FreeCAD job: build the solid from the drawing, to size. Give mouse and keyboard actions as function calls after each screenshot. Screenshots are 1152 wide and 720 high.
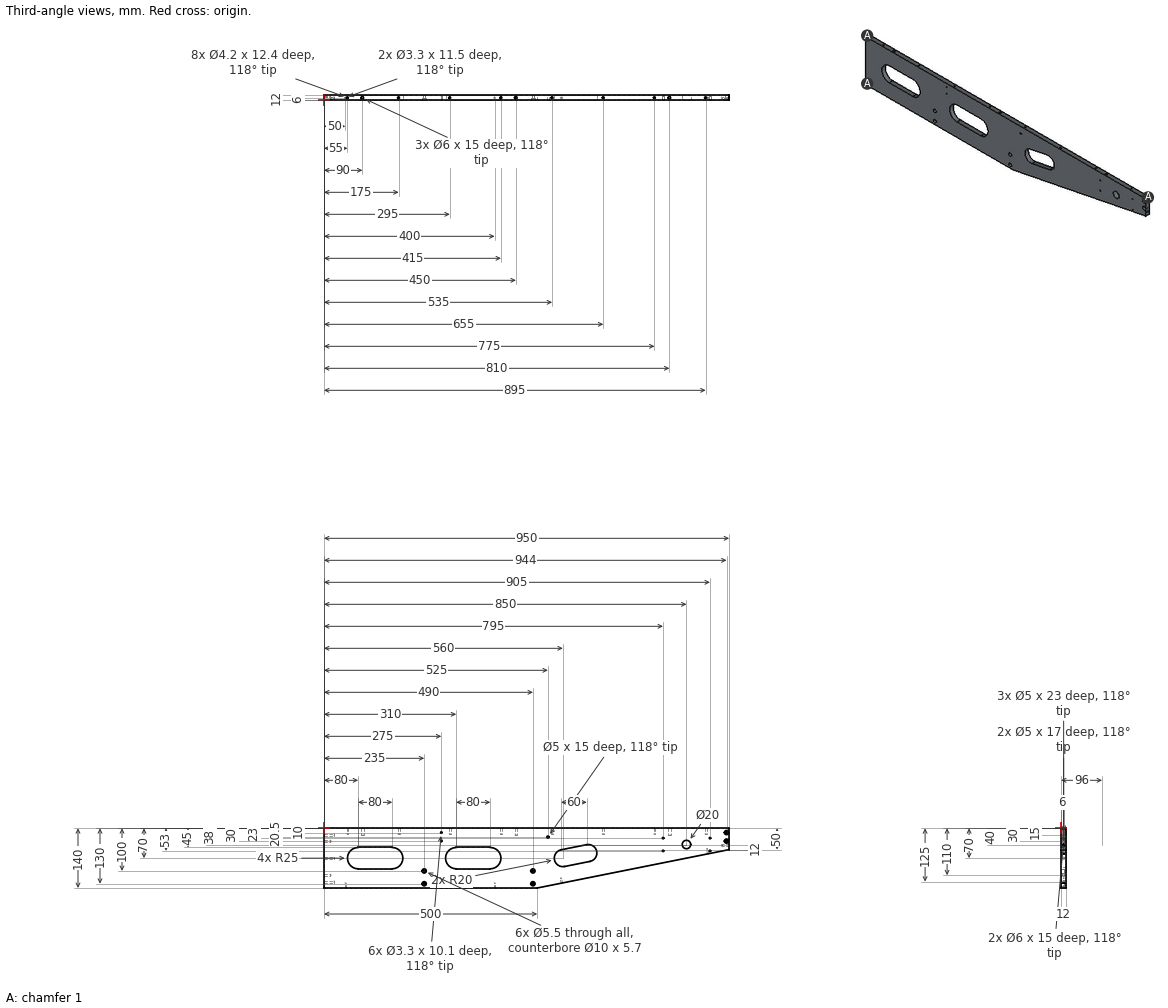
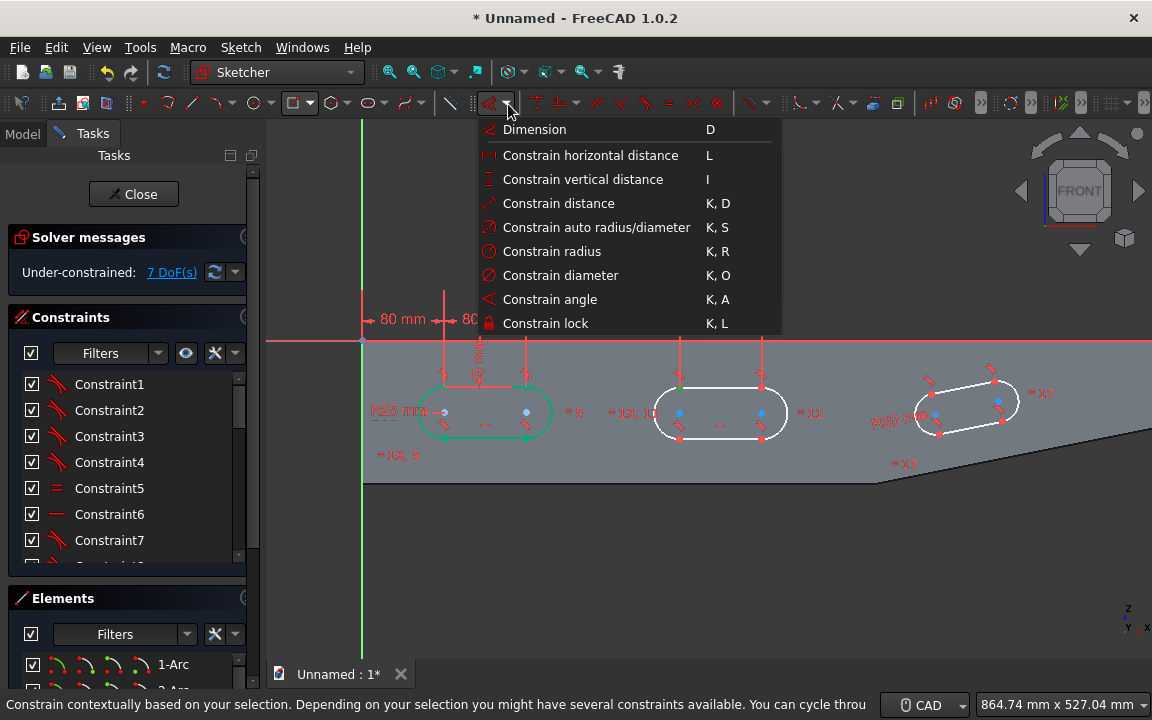
click(630, 179)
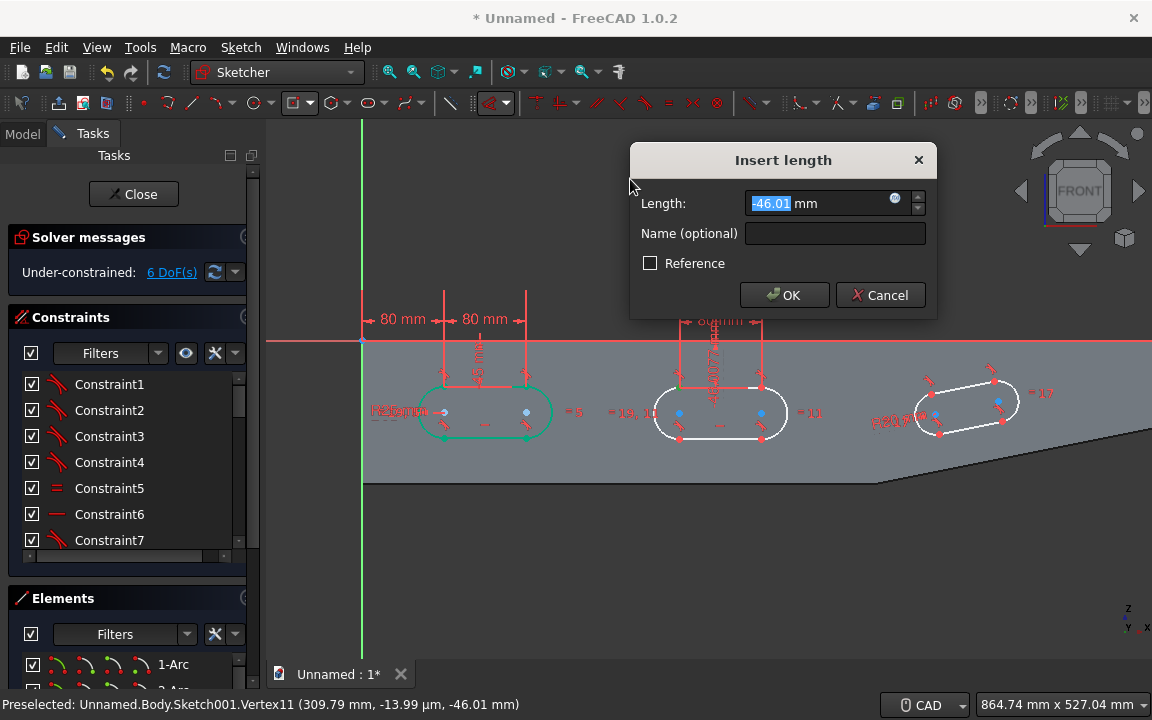
text(-45)
key(Return)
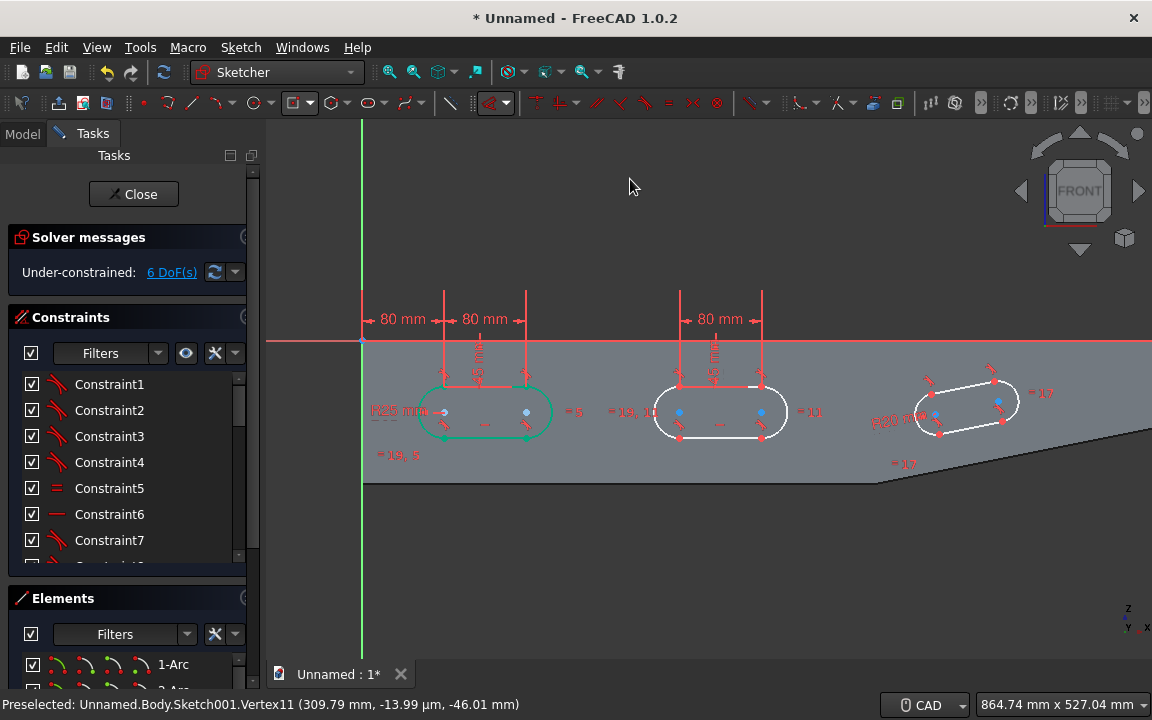
click(950, 390)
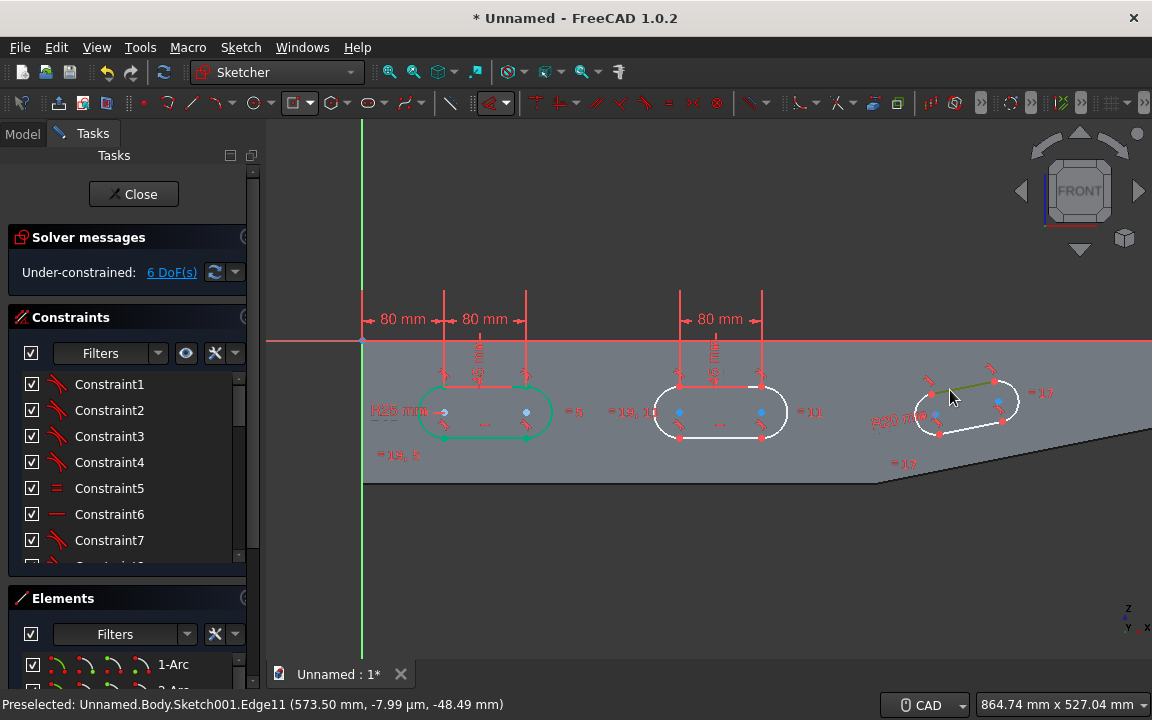
key(l)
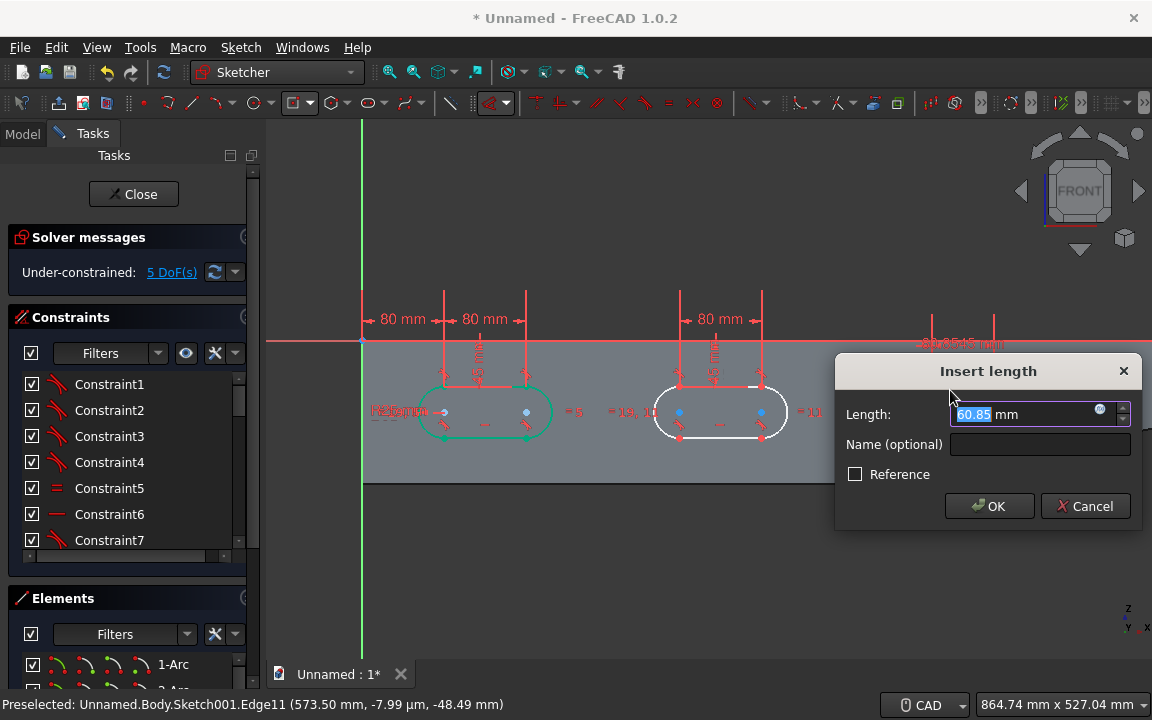
text(60)
key(Return)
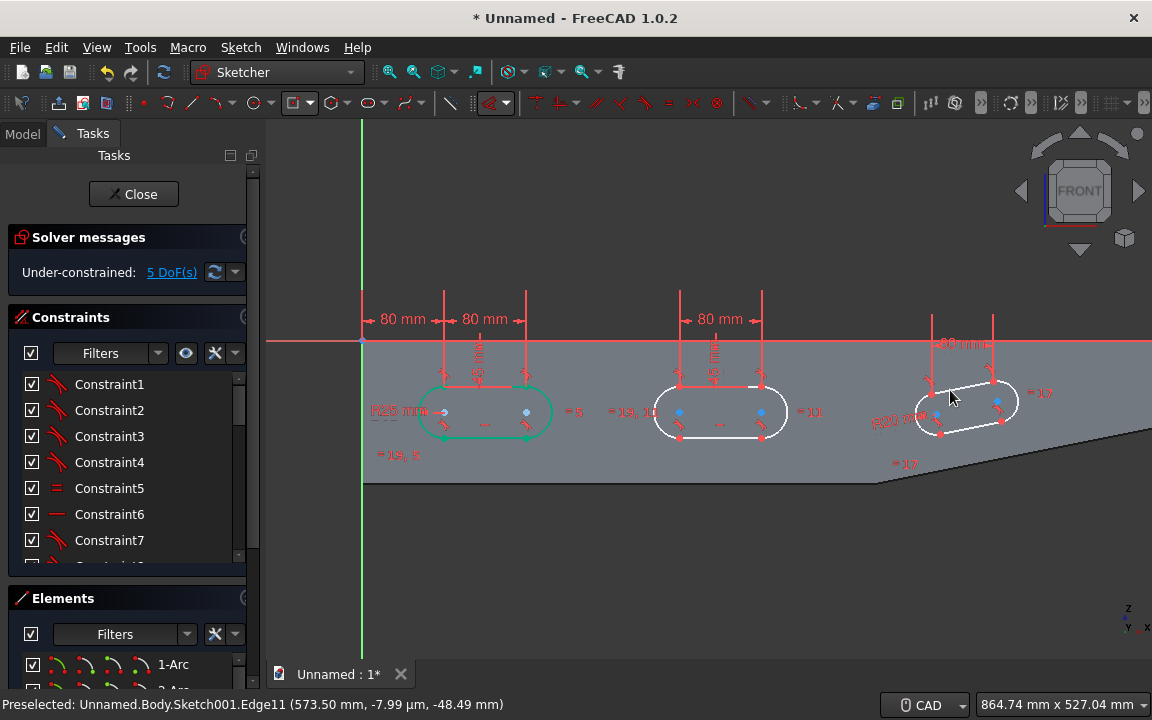
scroll(950, 390, up, 6)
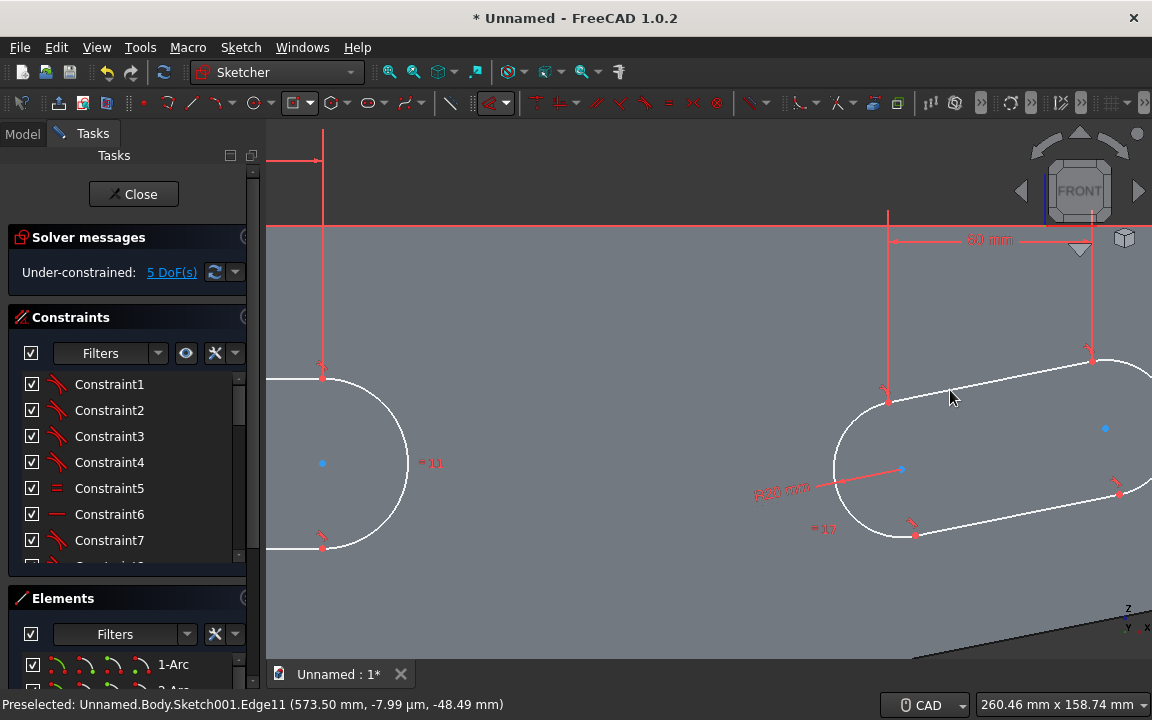
click(950, 390)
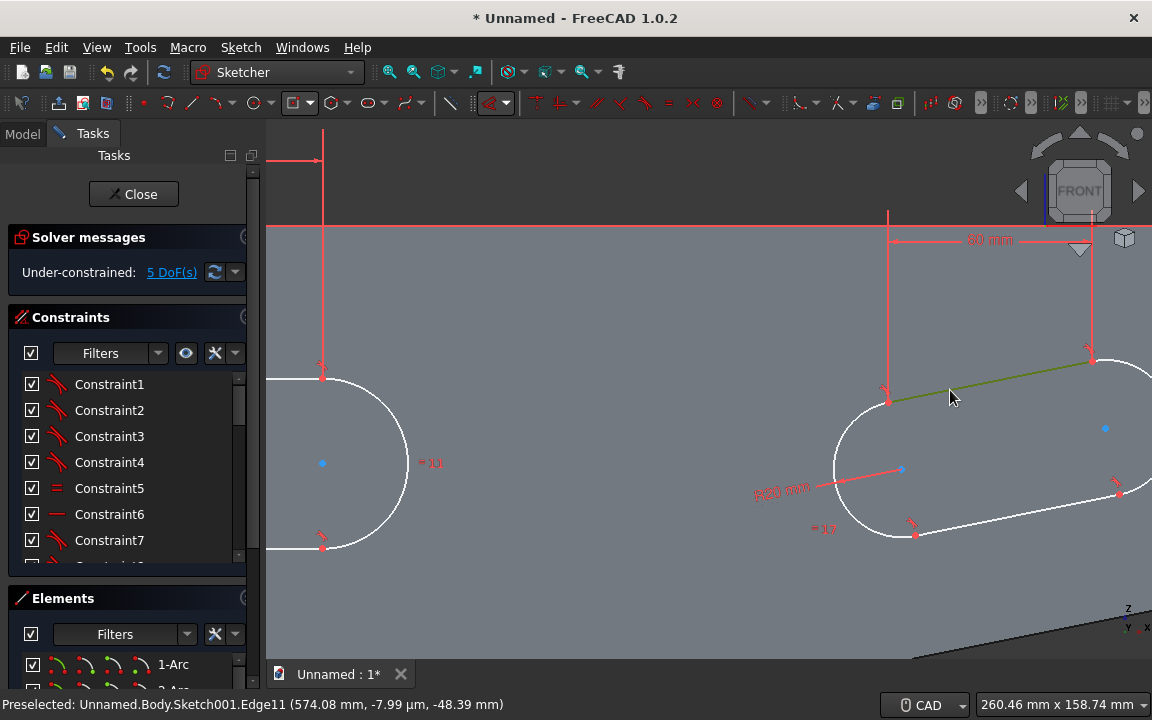
key(i)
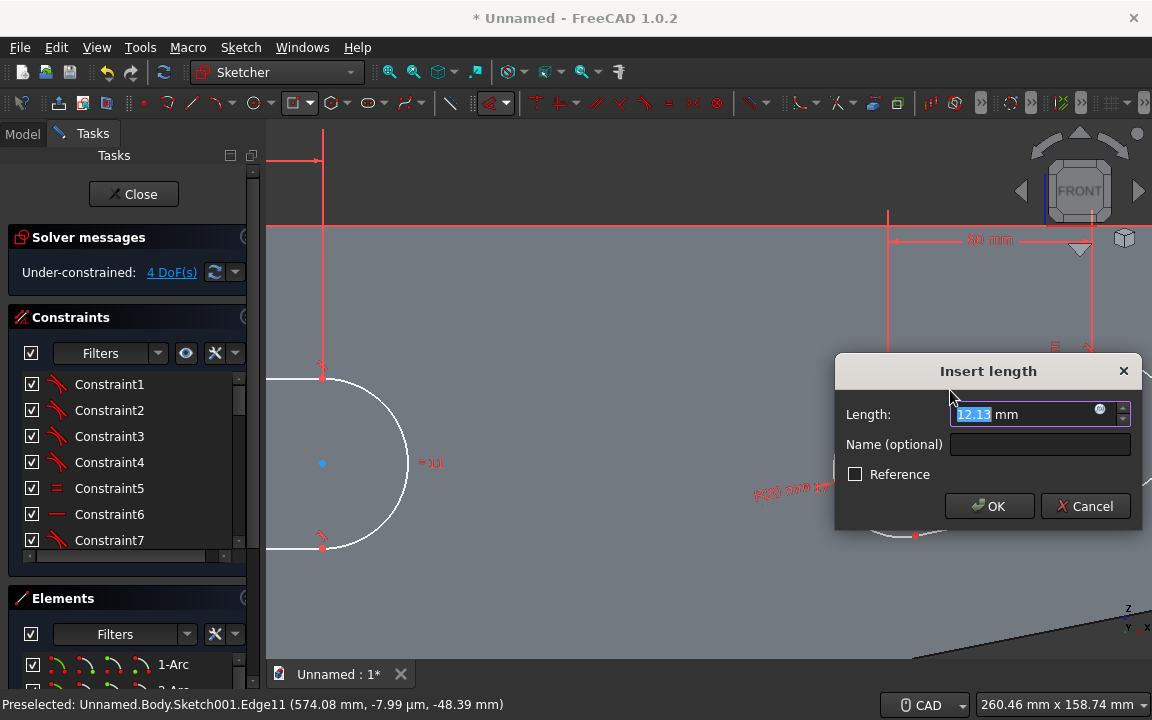
text(12)
key(Return)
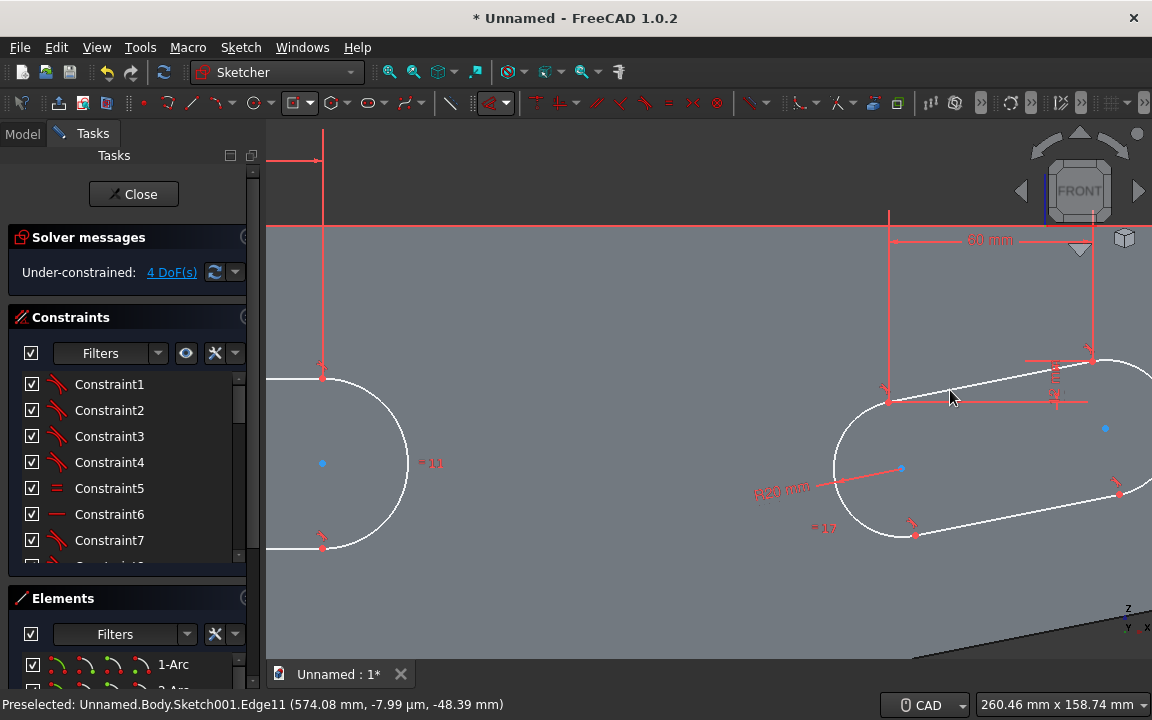
scroll(676, 389, down, 9)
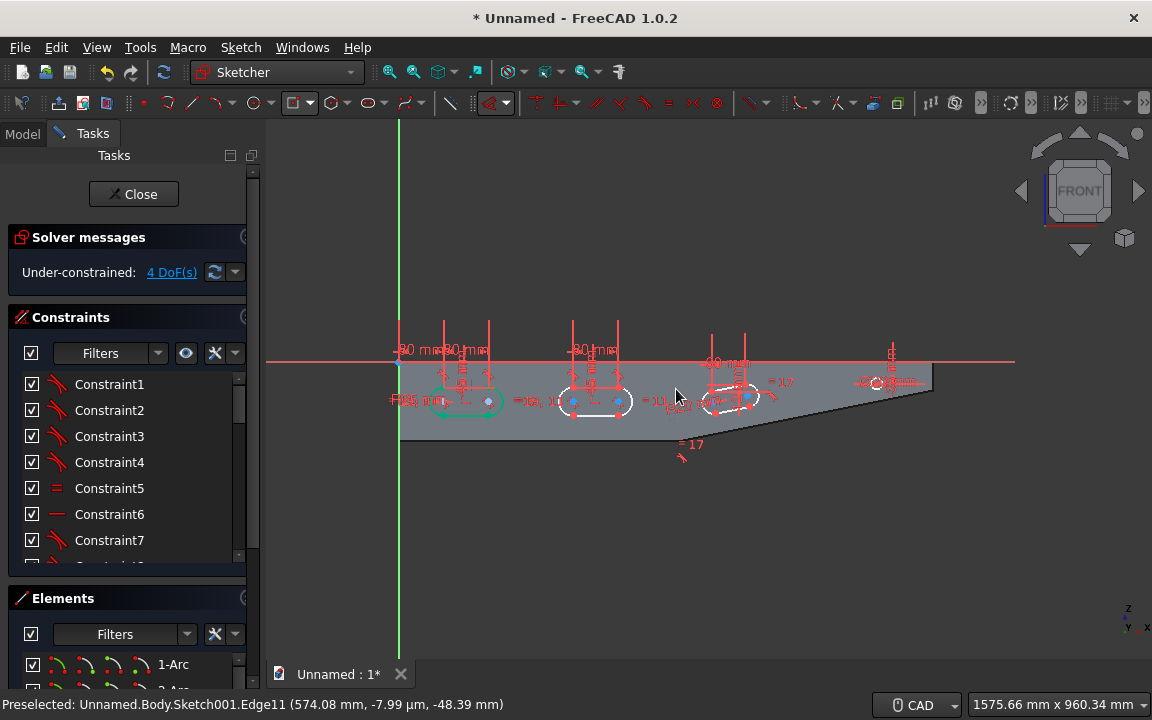
click(714, 403)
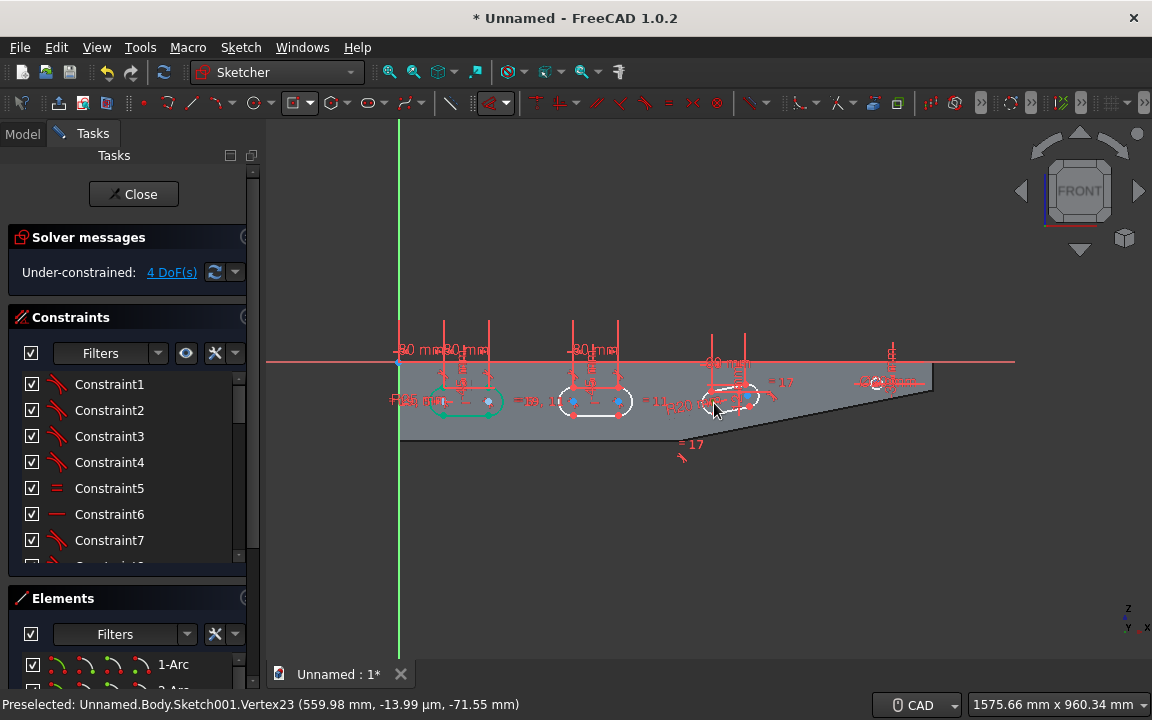
key(i)